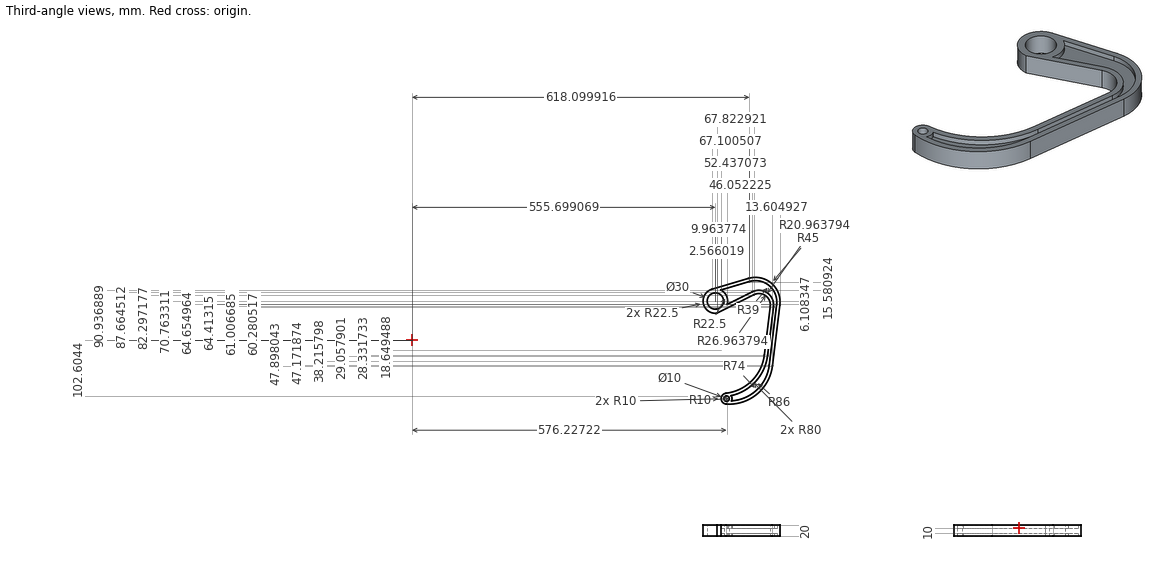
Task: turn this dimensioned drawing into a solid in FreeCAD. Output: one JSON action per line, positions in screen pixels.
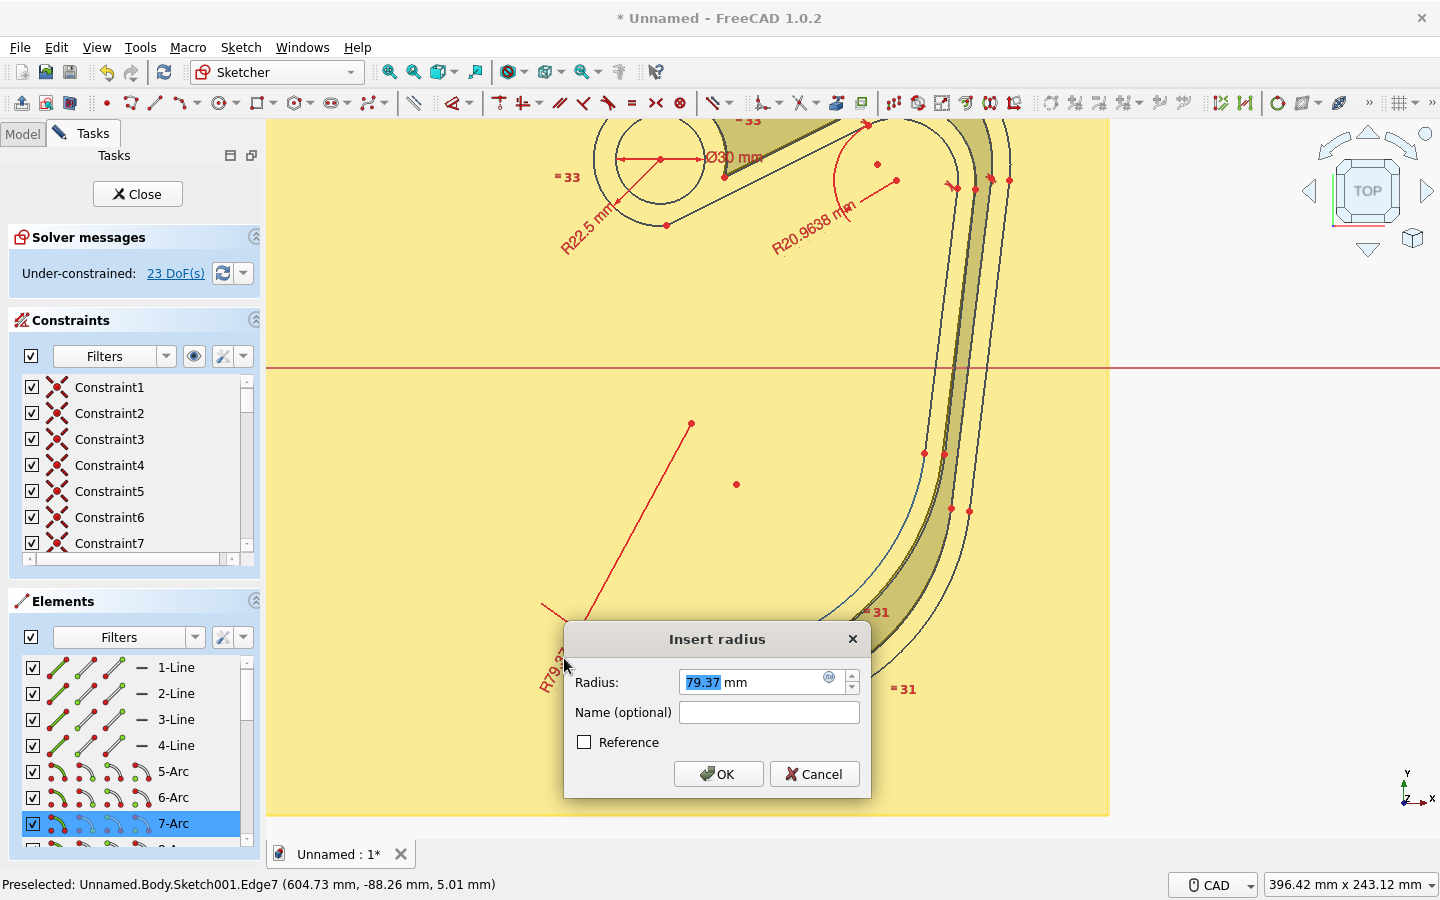
{"action": "type", "text": "80"}
{"action": "key", "text": "Return"}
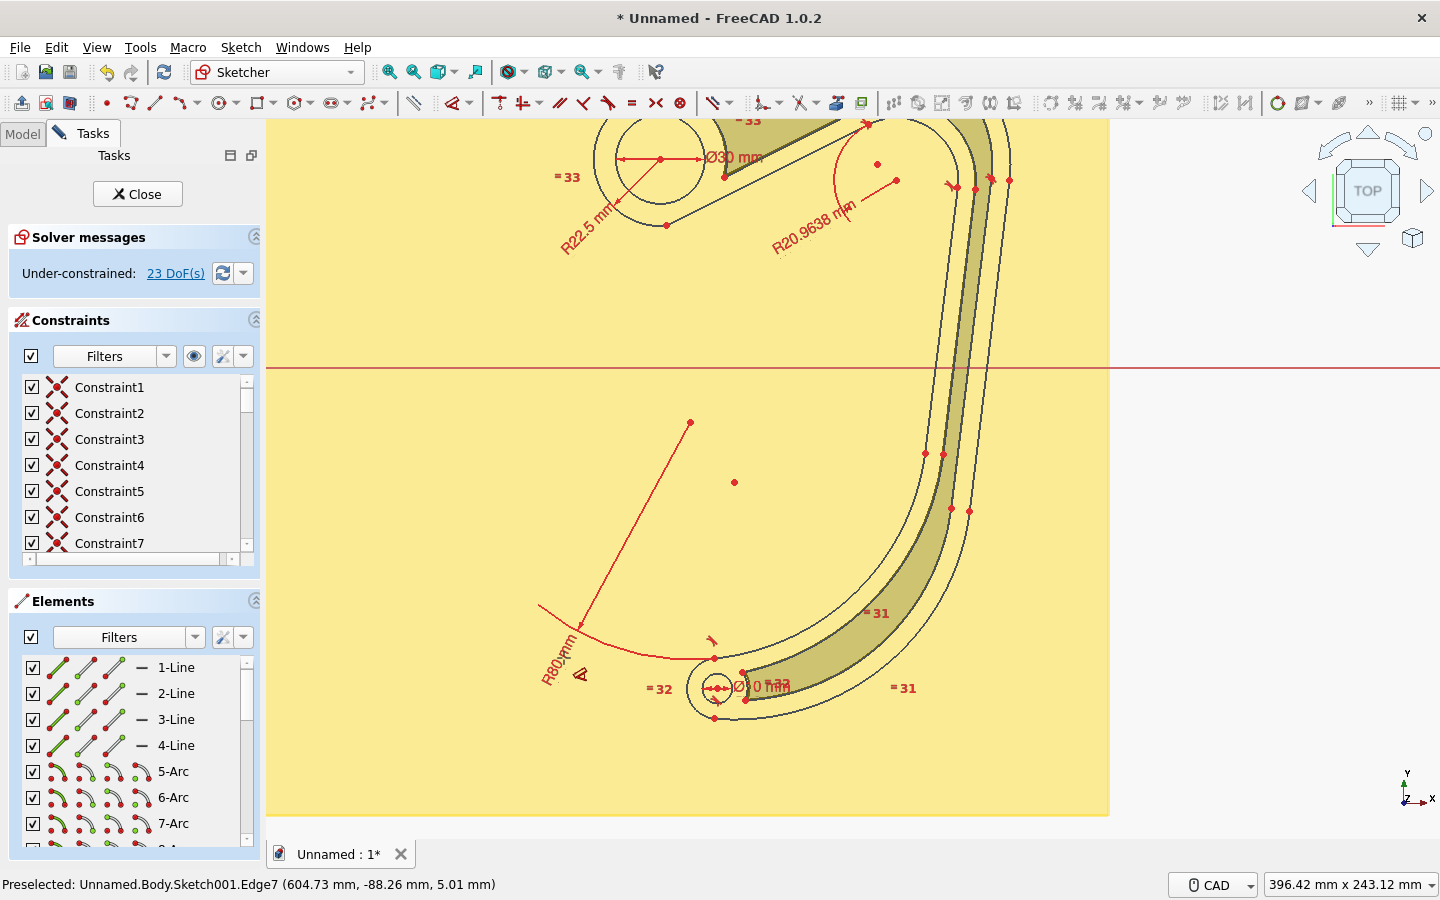
{"action": "scroll", "coordinate": [692, 672], "scroll_direction": "up", "scroll_amount": 2}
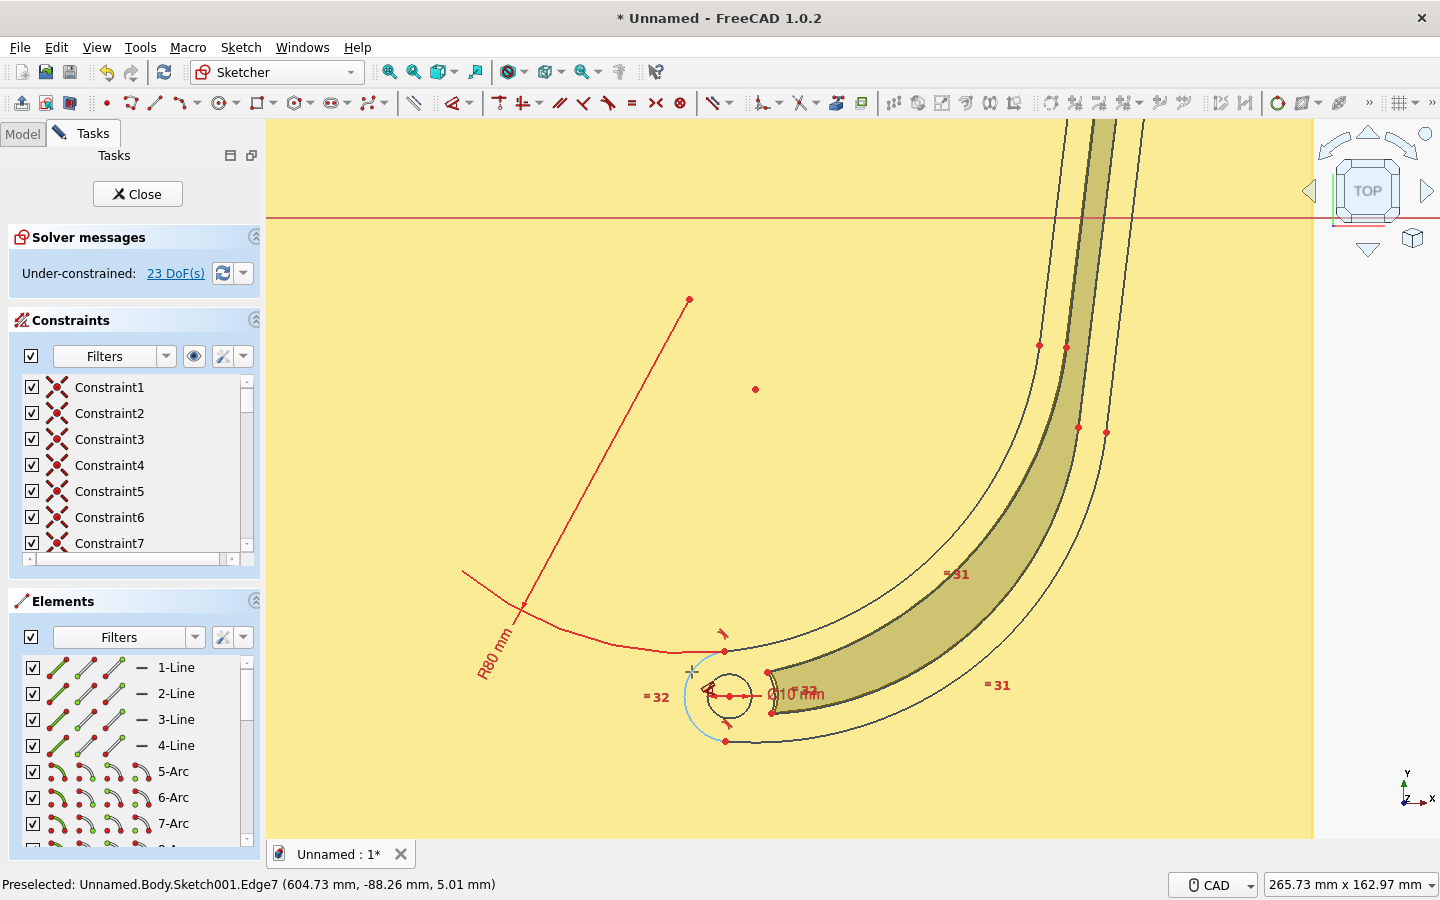
{"action": "left_click", "coordinate": [692, 672]}
{"action": "left_click", "coordinate": [665, 655]}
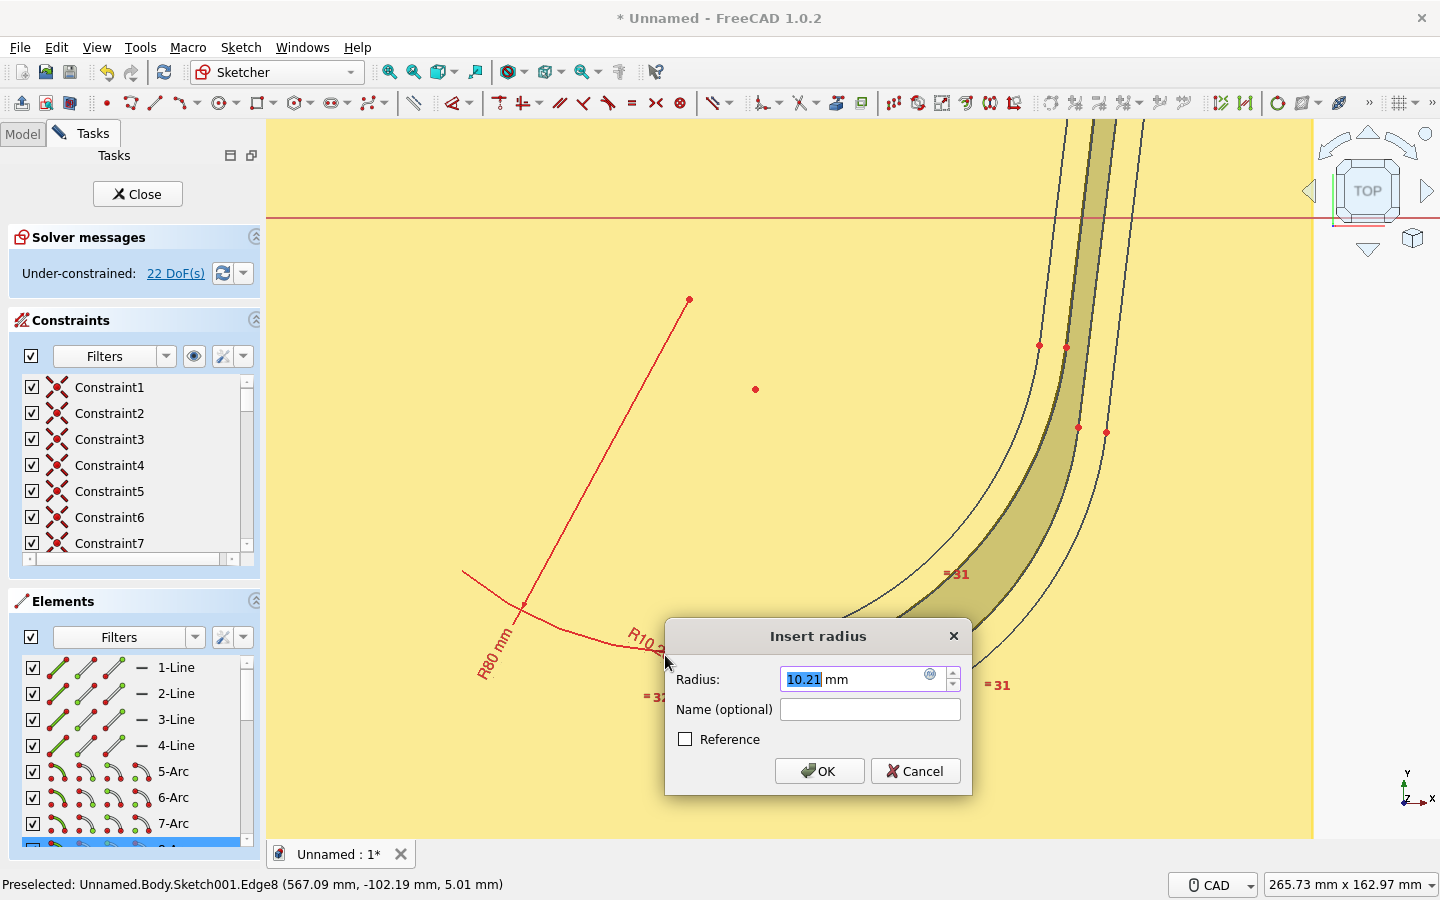
{"action": "type", "text": "10"}
{"action": "key", "text": "Return"}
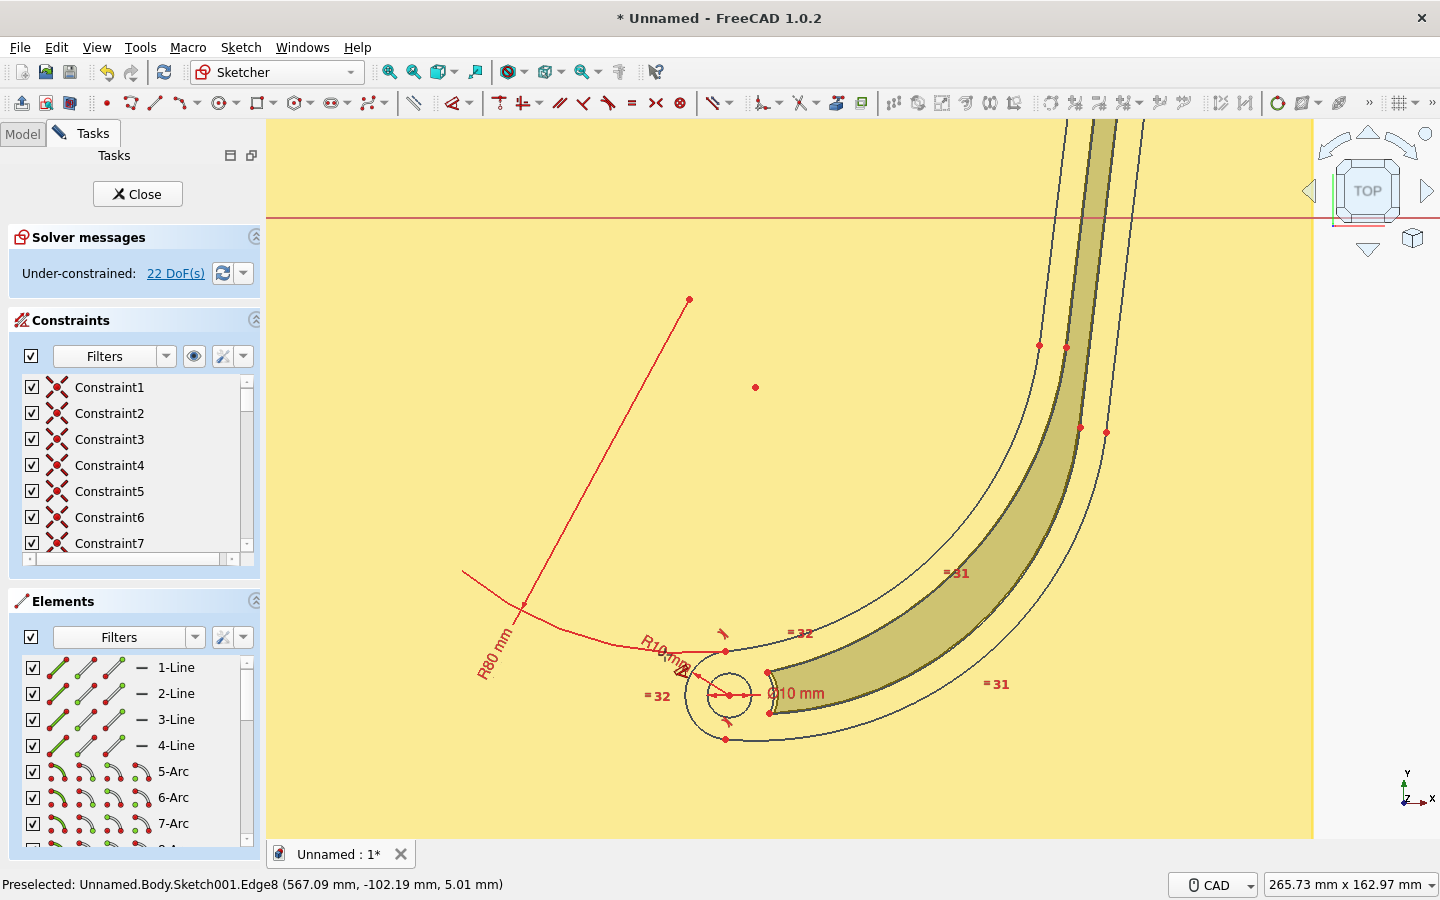
{"action": "scroll", "coordinate": [727, 682], "scroll_direction": "down", "scroll_amount": 4}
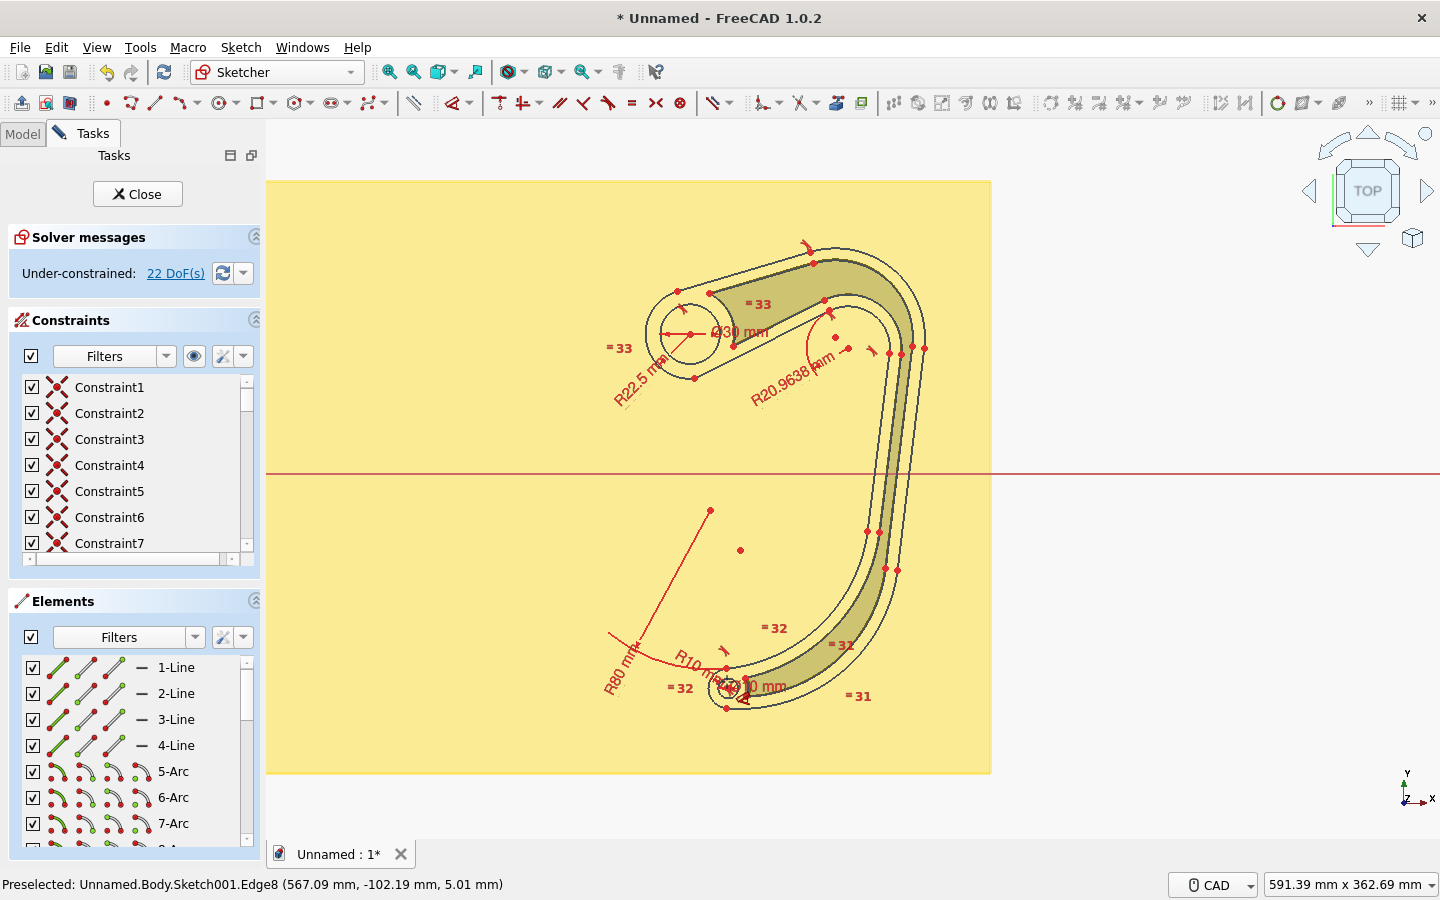
{"action": "left_click", "coordinate": [915, 297]}
{"action": "left_click", "coordinate": [943, 282]}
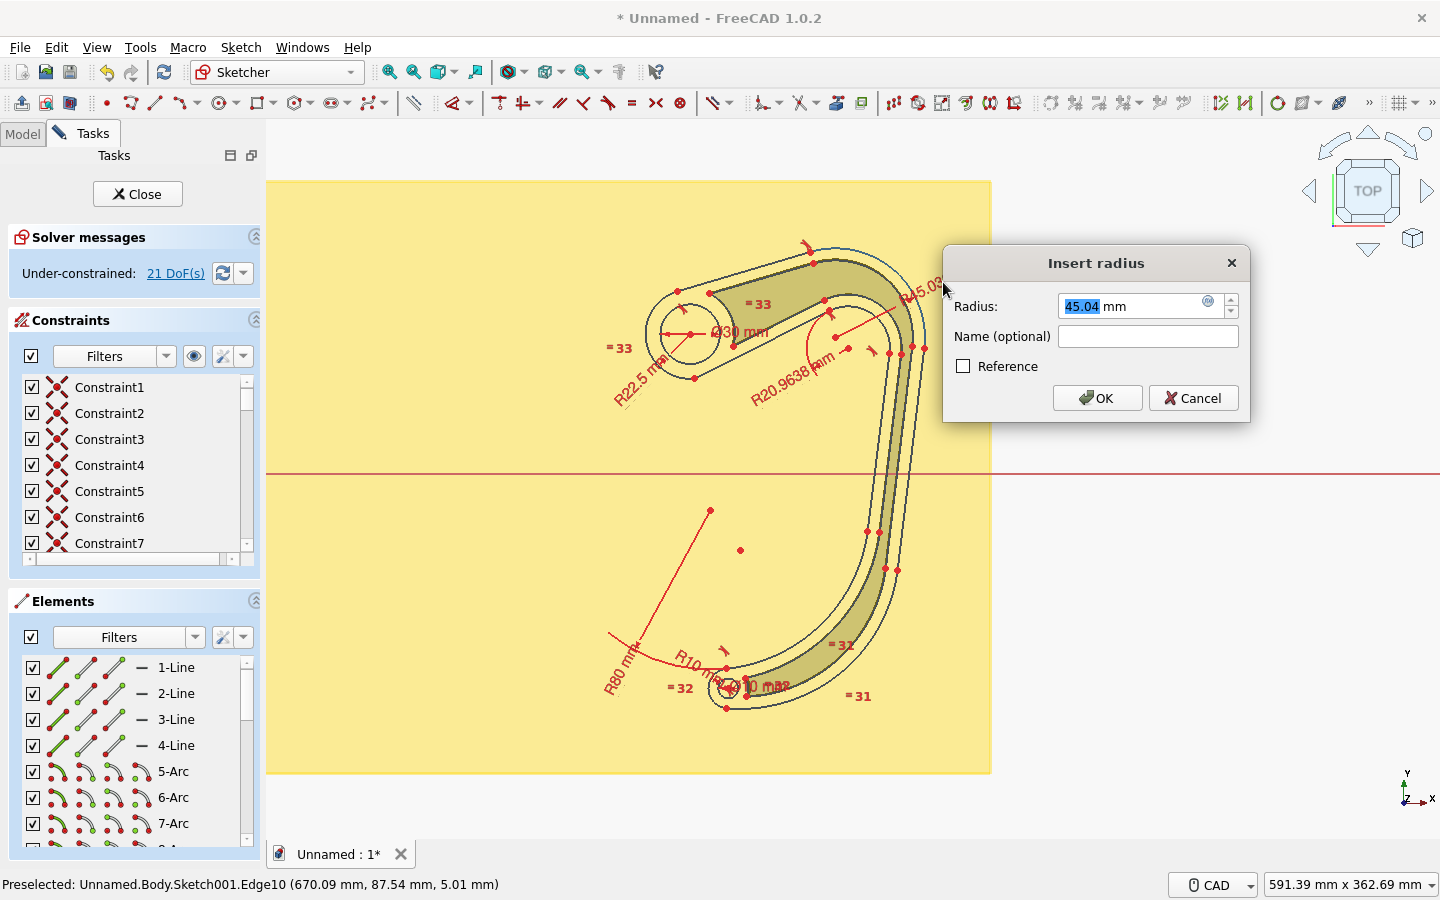
{"action": "type", "text": "45"}
{"action": "key", "text": "Return"}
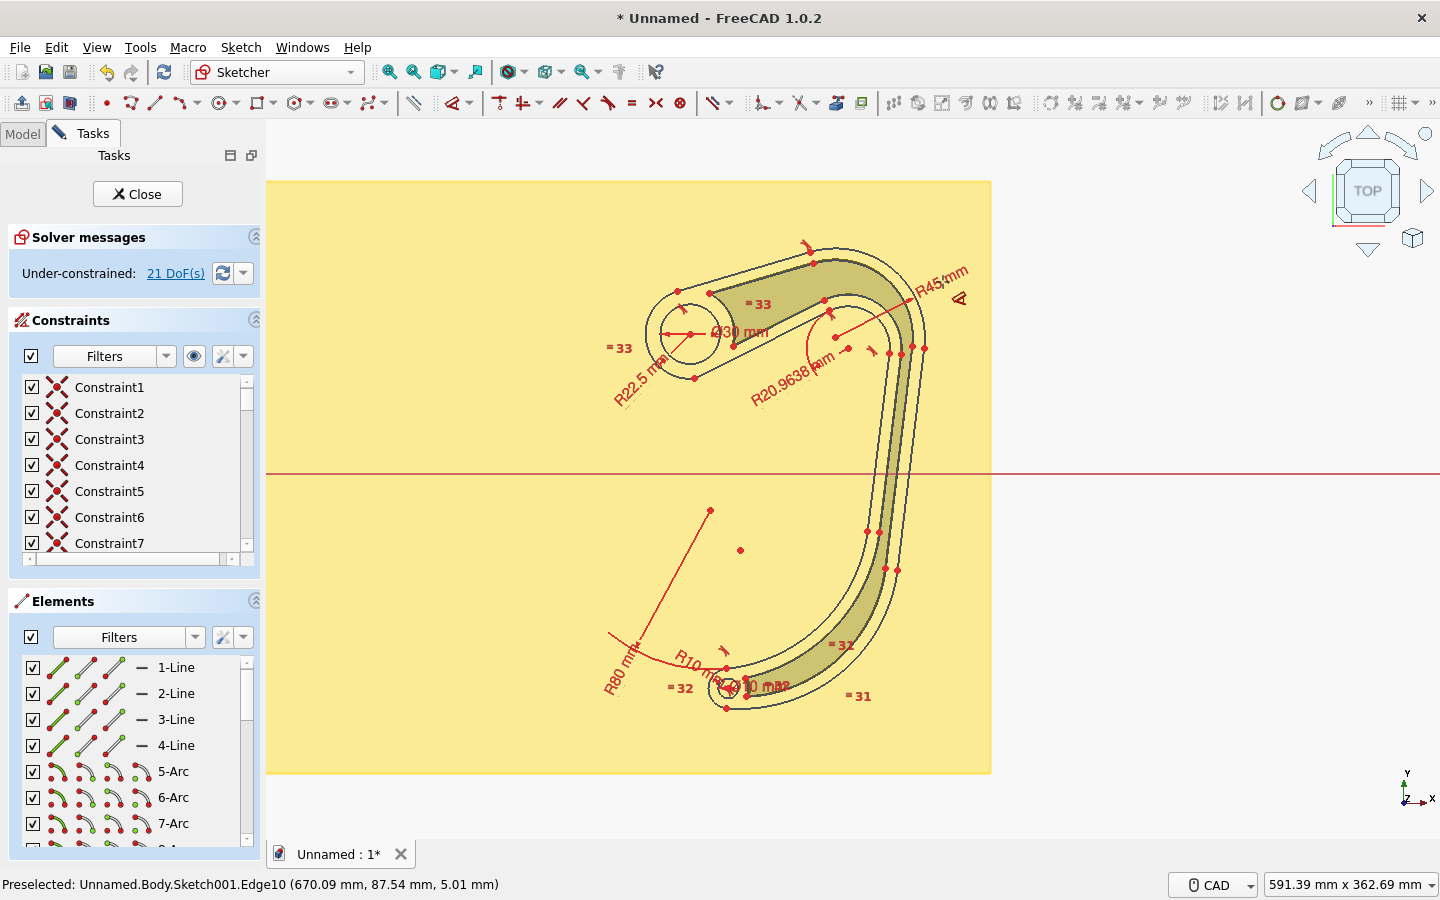
{"action": "left_click", "coordinate": [904, 303]}
{"action": "left_click", "coordinate": [944, 341]}